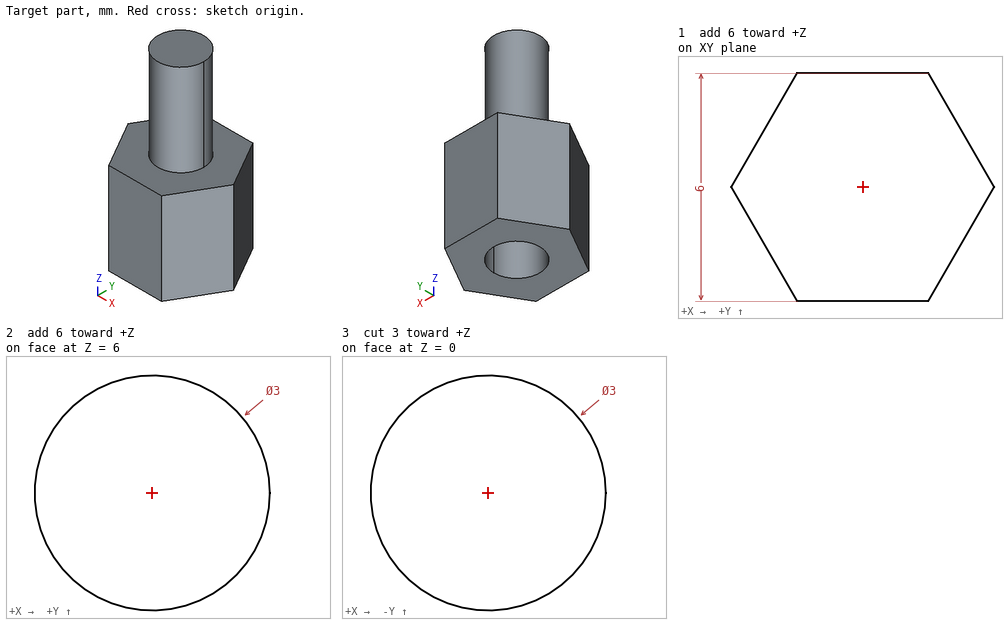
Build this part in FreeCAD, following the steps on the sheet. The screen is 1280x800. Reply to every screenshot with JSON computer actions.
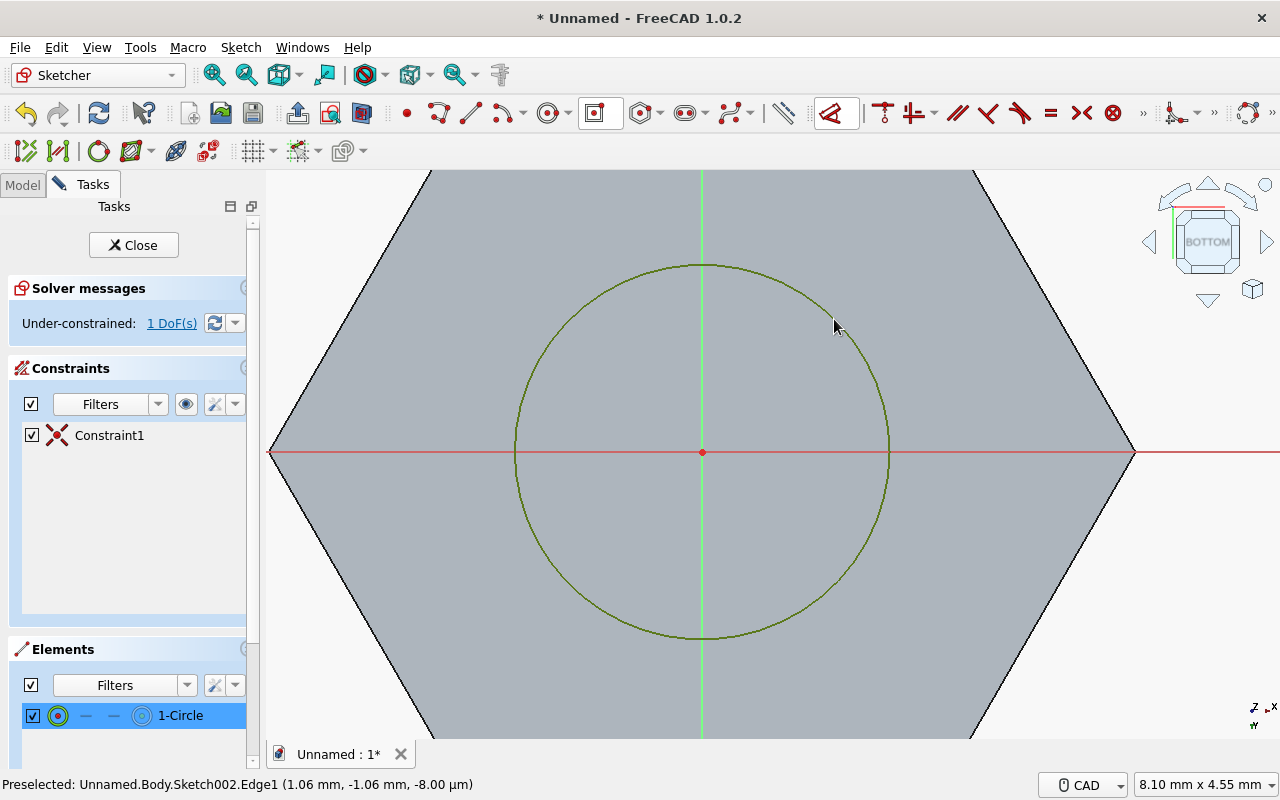
{"action": "left_click", "coordinate": [854, 114]}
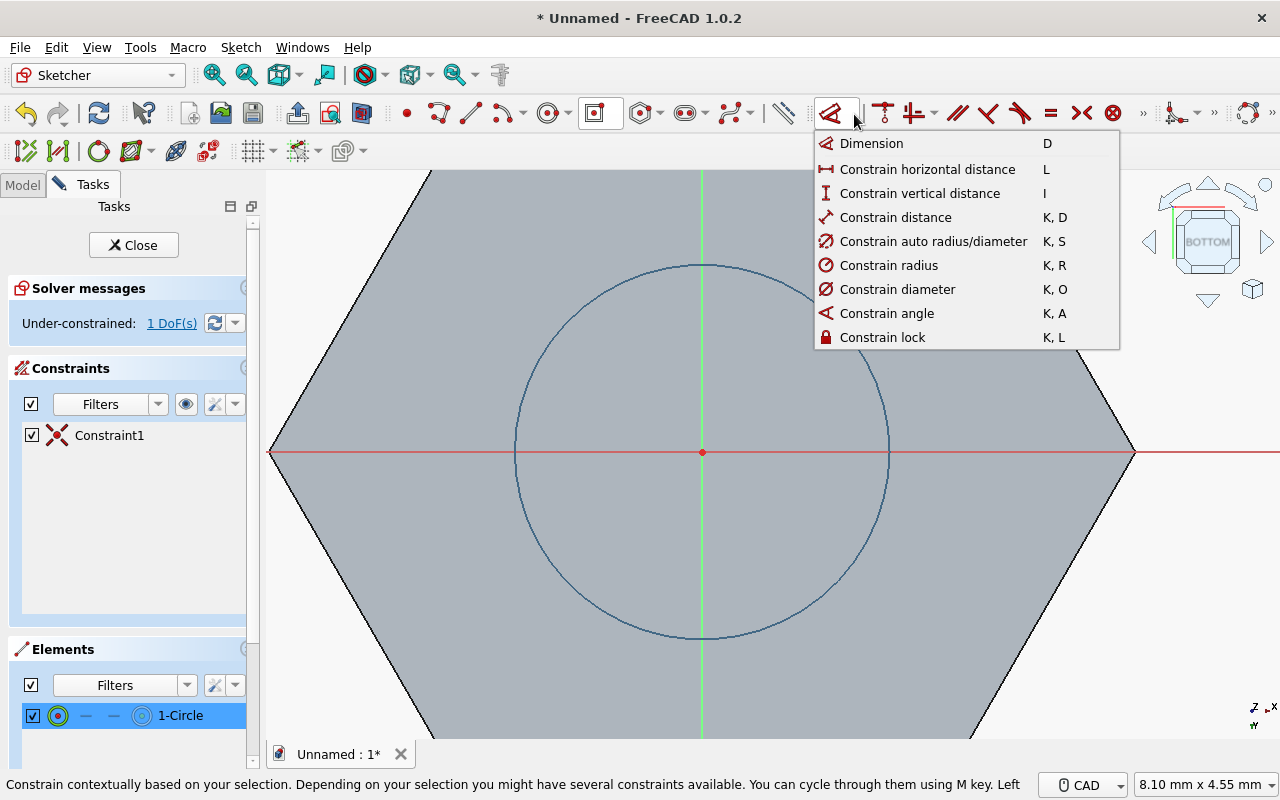
{"action": "left_click", "coordinate": [967, 289]}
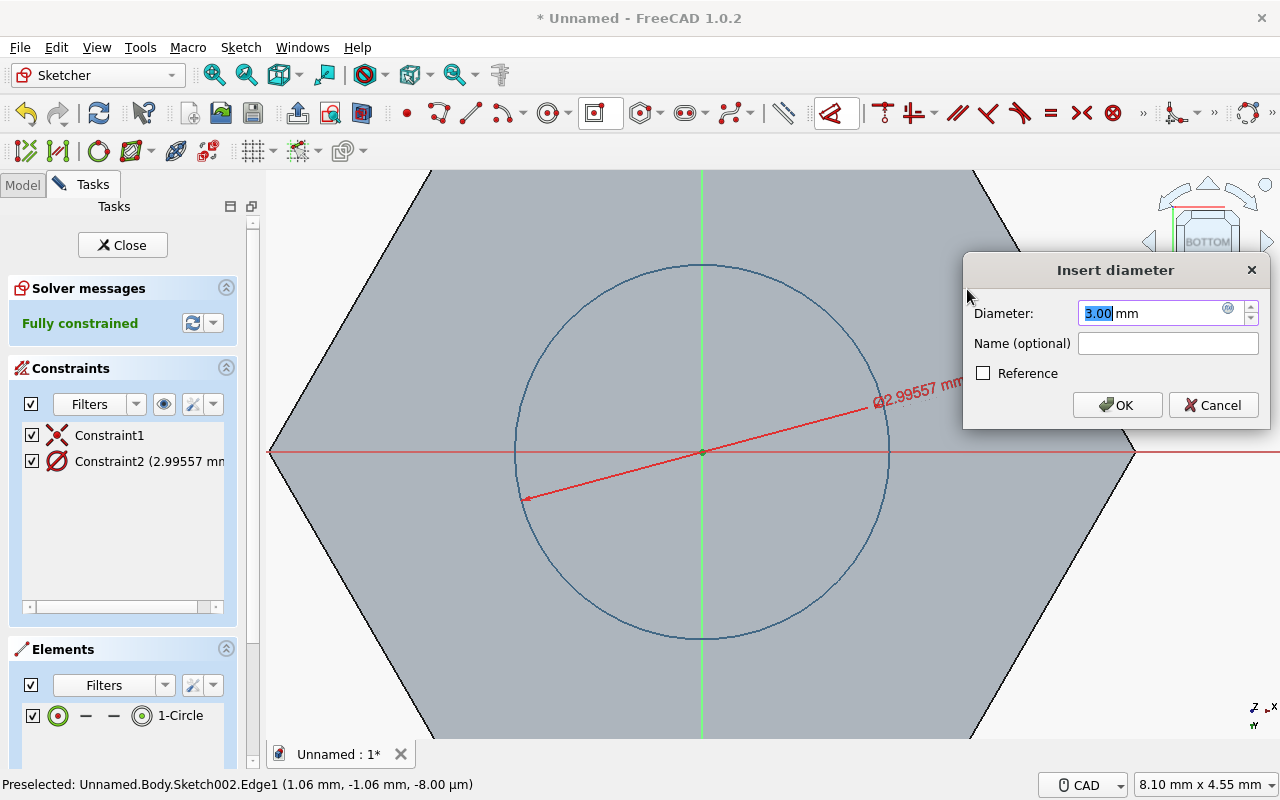
{"action": "type", "text": "3"}
{"action": "key", "text": "Return"}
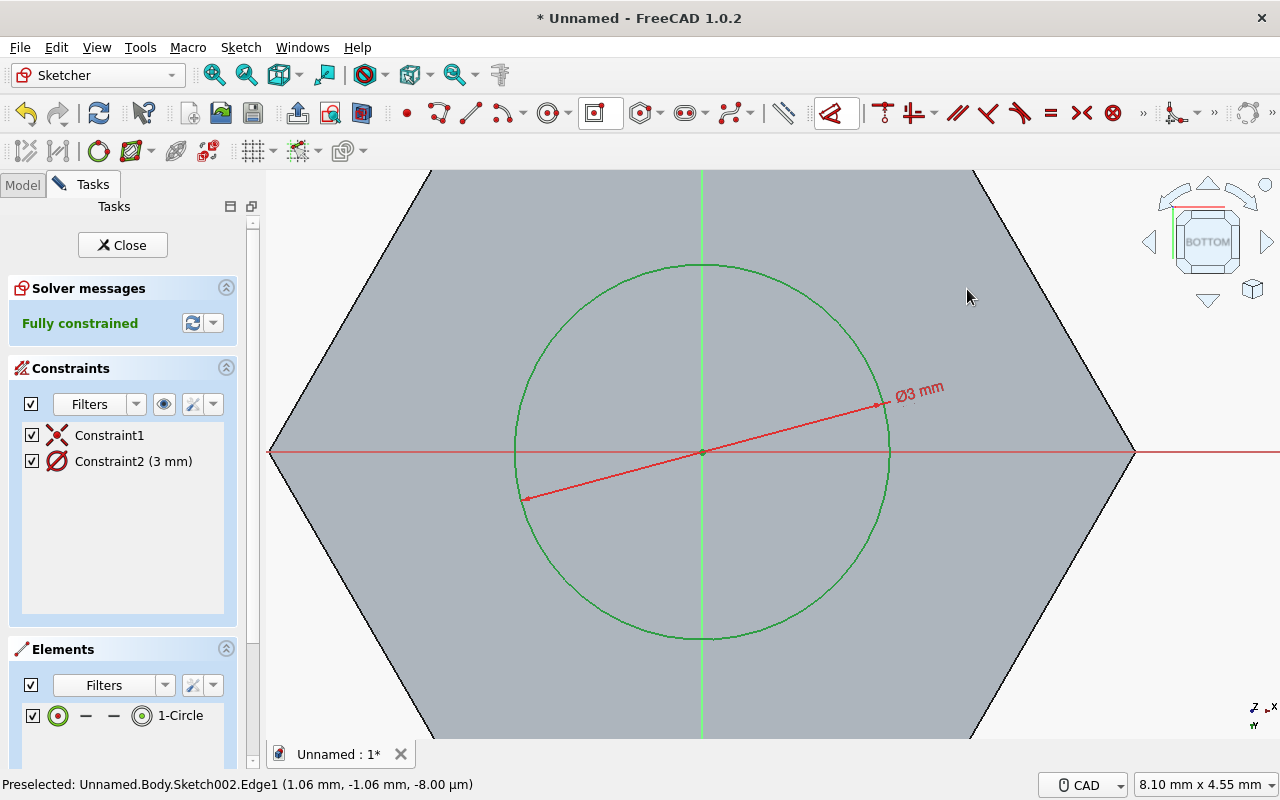
{"action": "left_click", "coordinate": [123, 245]}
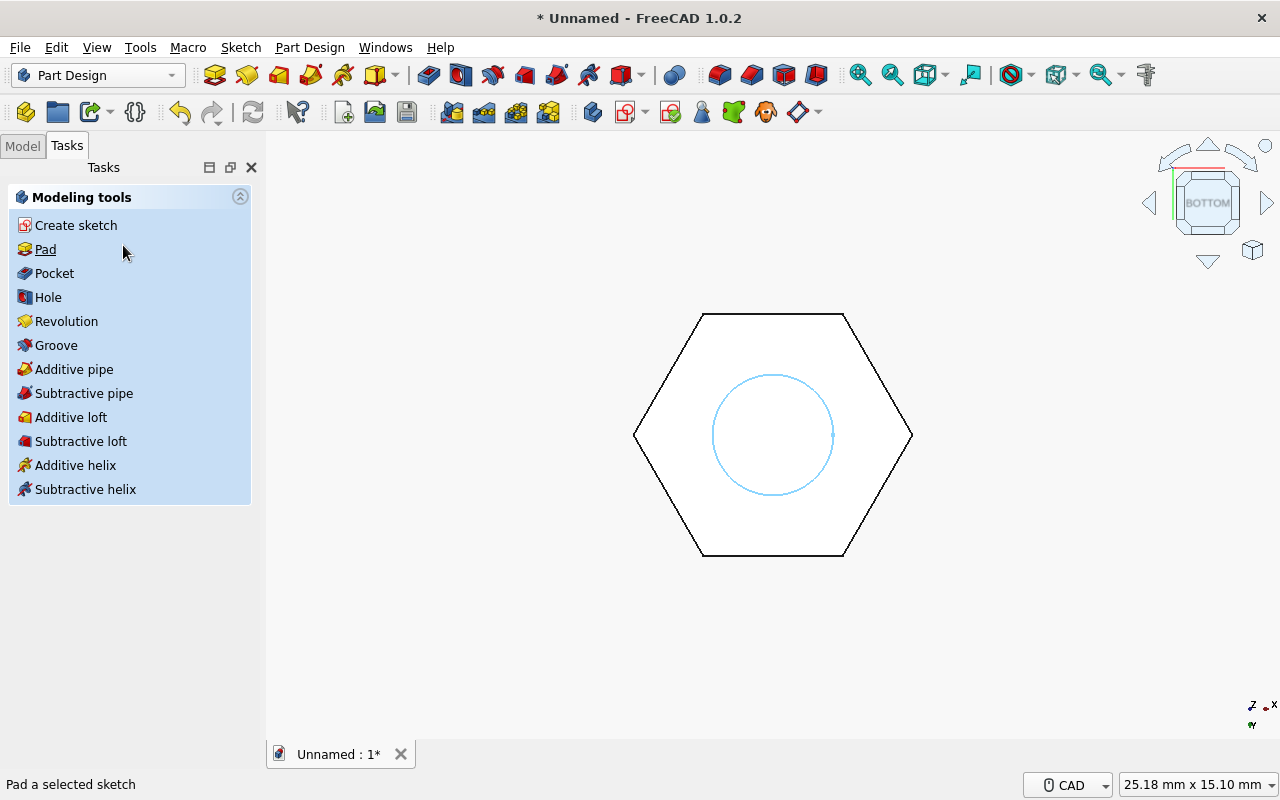
{"action": "left_click", "coordinate": [430, 76]}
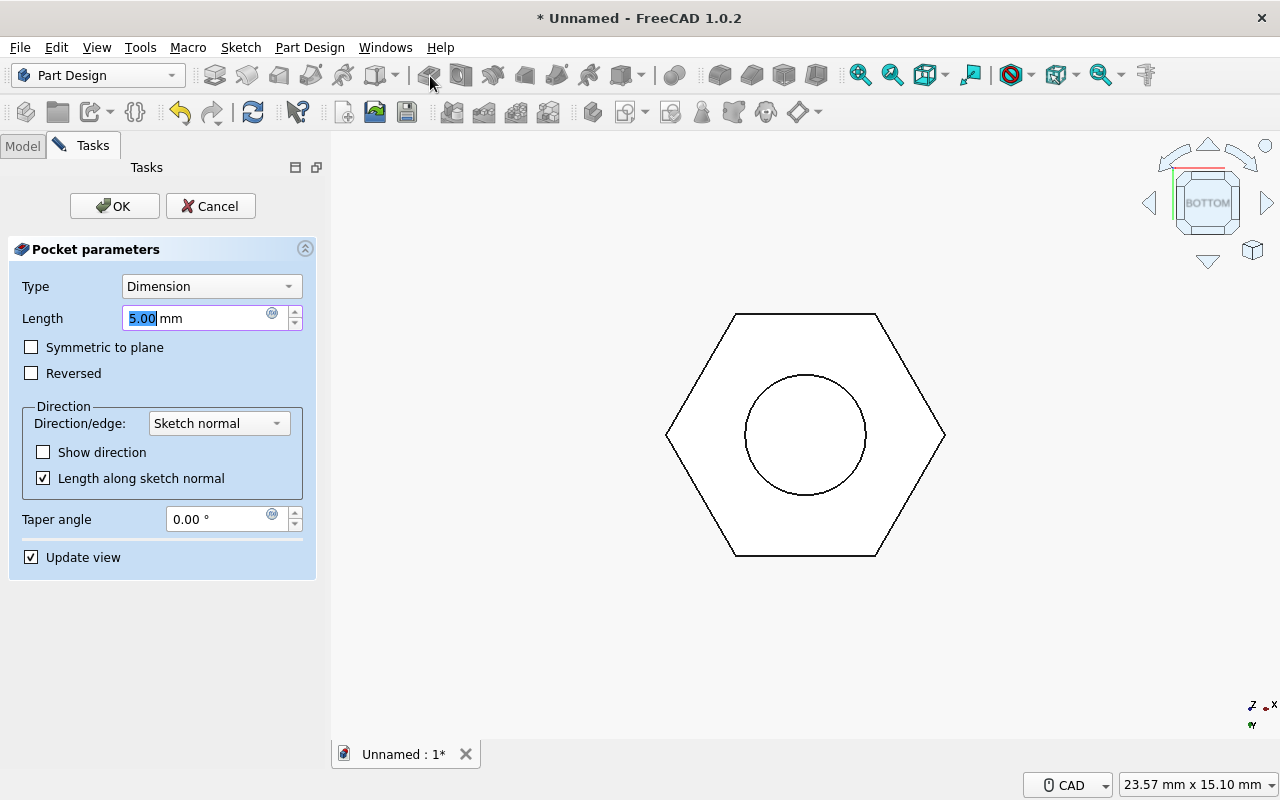
{"action": "type", "text": "3"}
{"action": "key", "text": "Tab"}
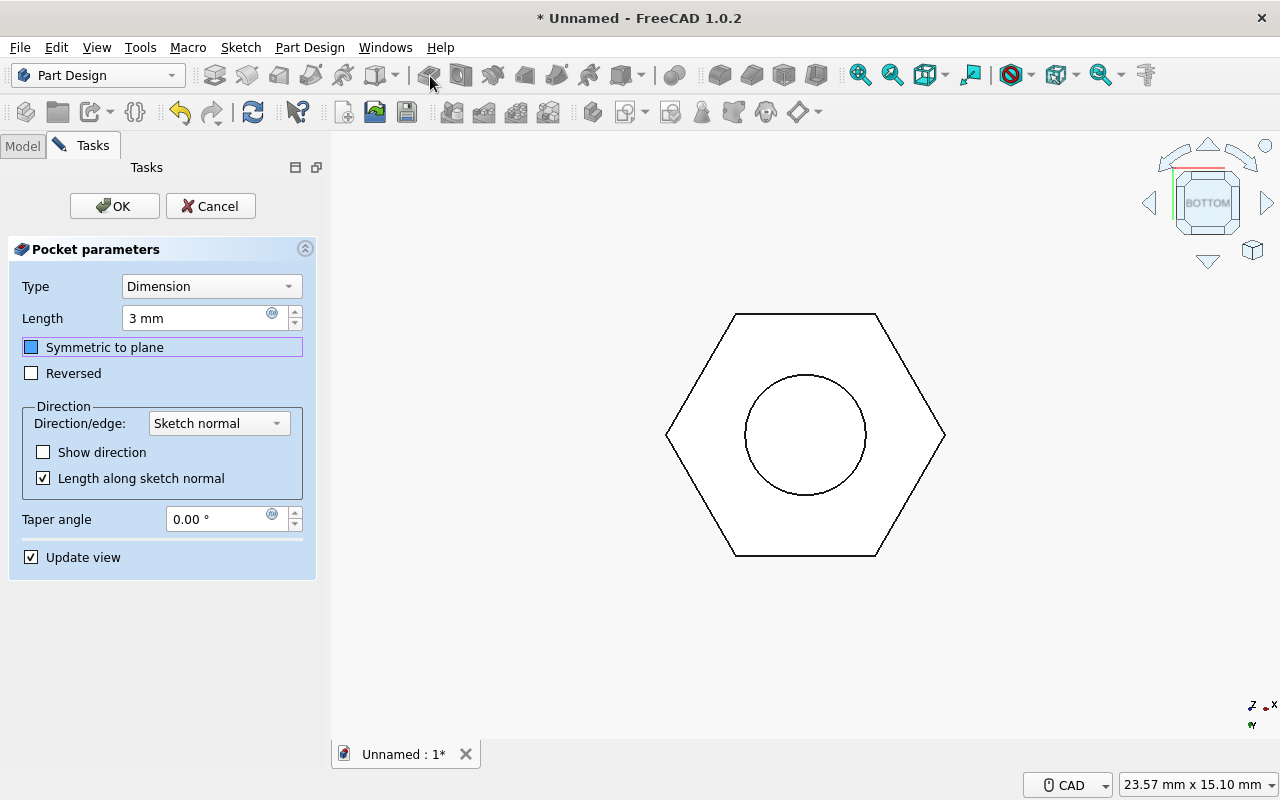
{"action": "left_click", "coordinate": [115, 206]}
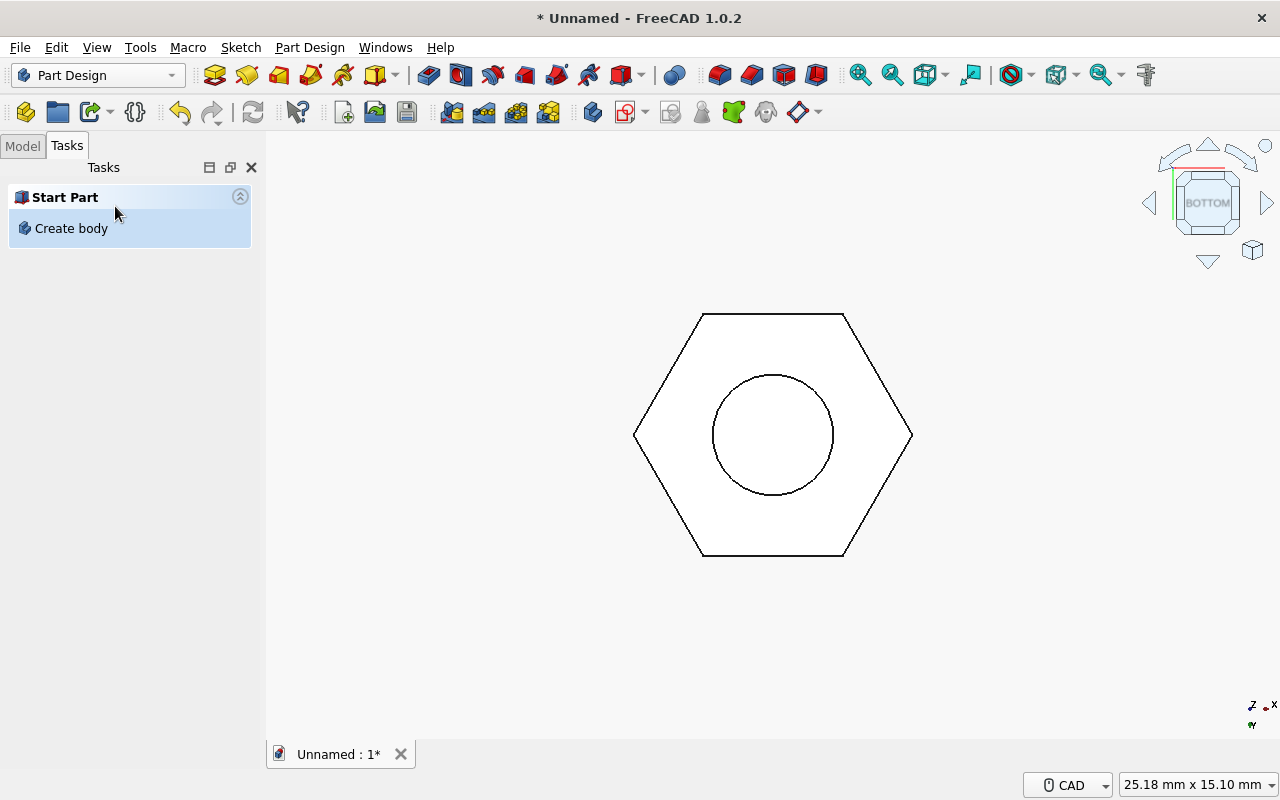
{"action": "key", "text": "0"}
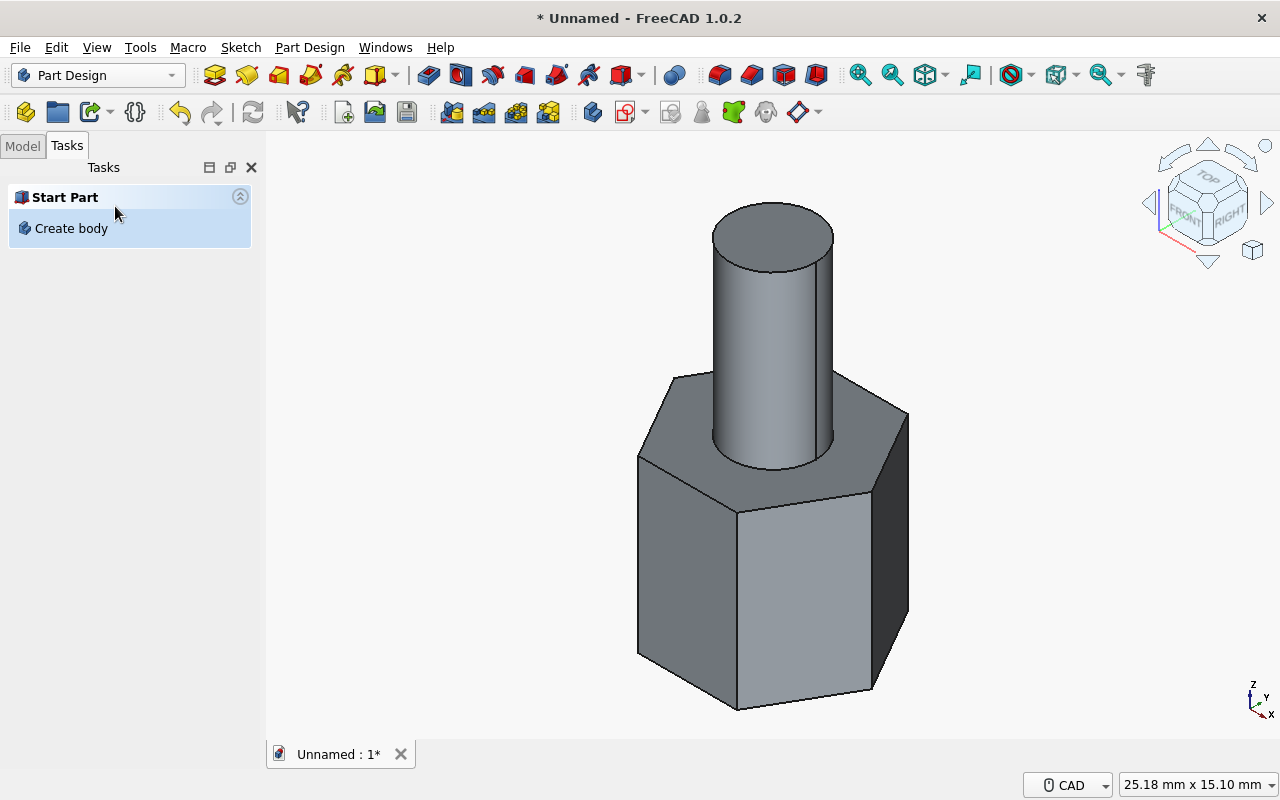
{"action": "key", "text": "v f"}